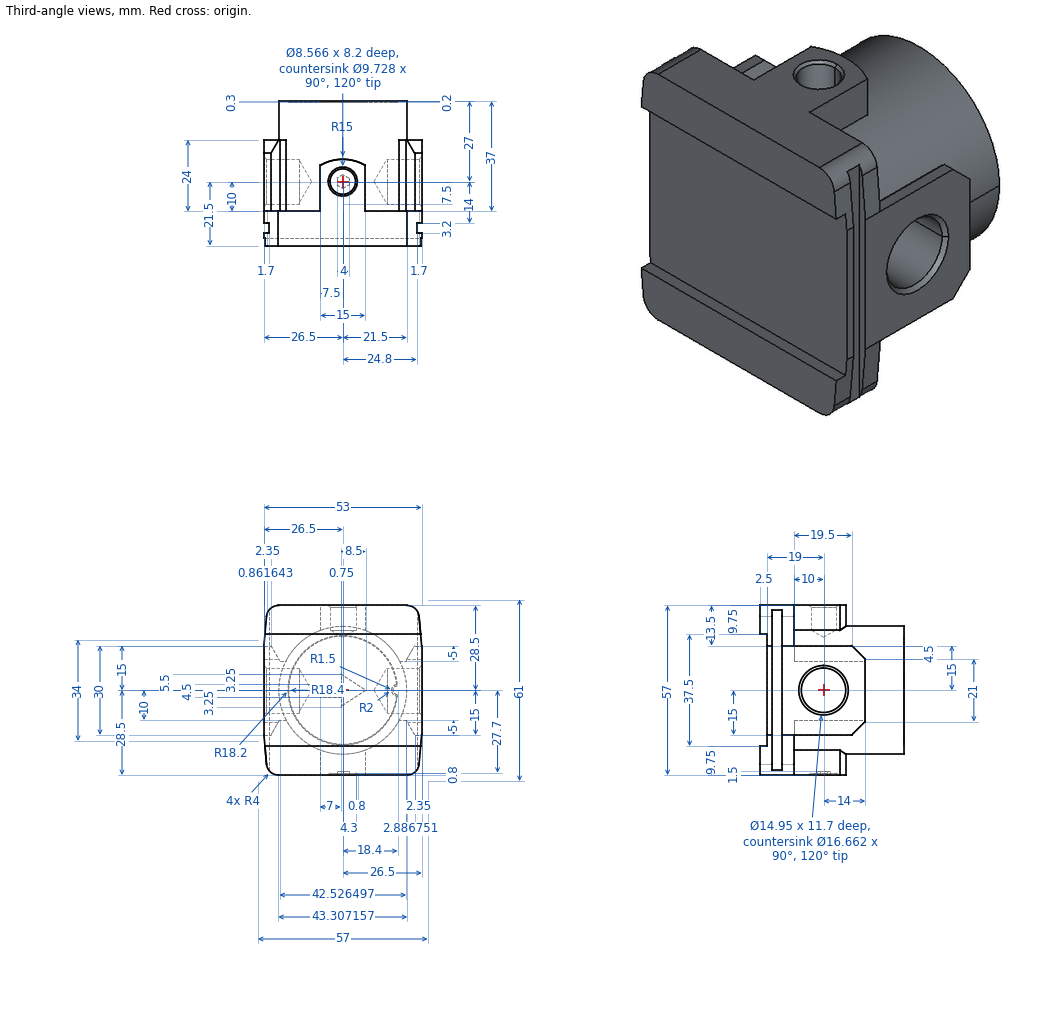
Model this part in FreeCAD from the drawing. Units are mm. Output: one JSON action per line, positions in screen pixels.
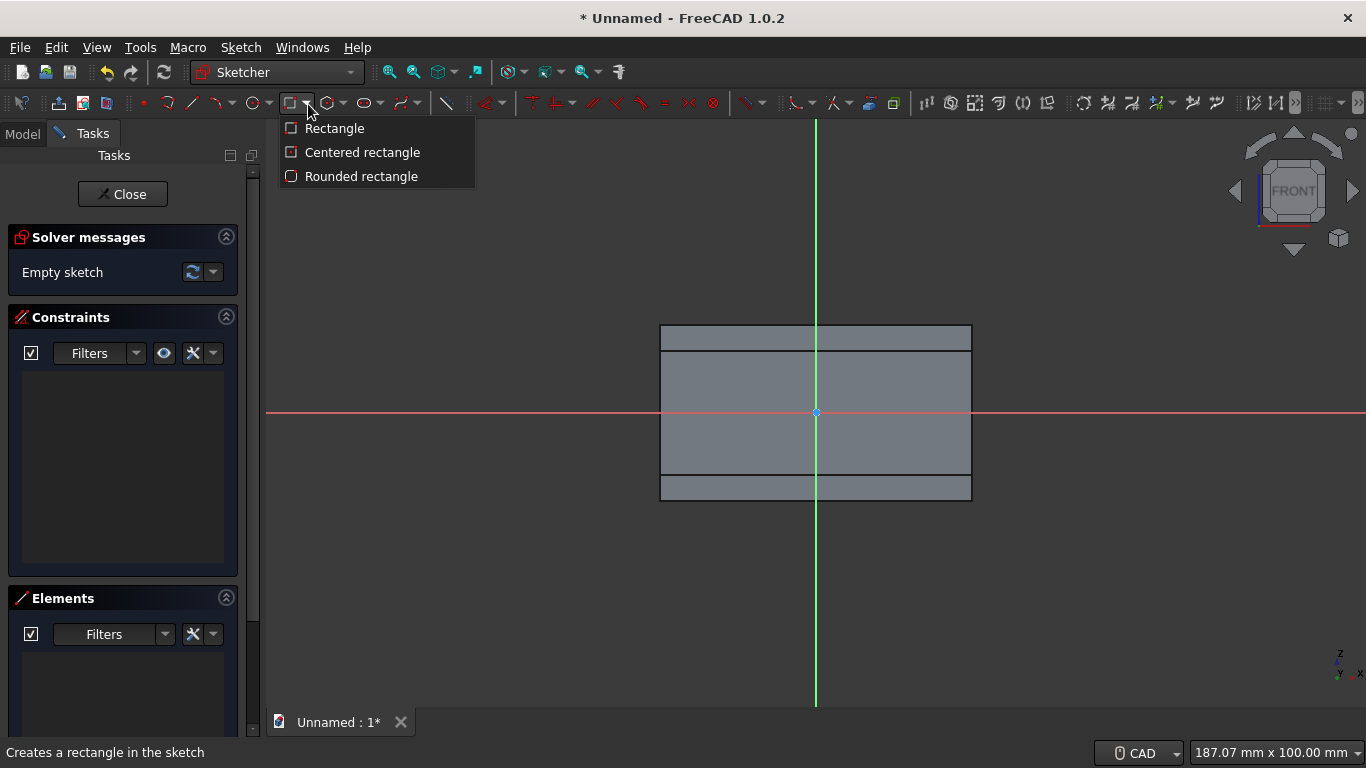
{"action": "left_click", "coordinate": [378, 152]}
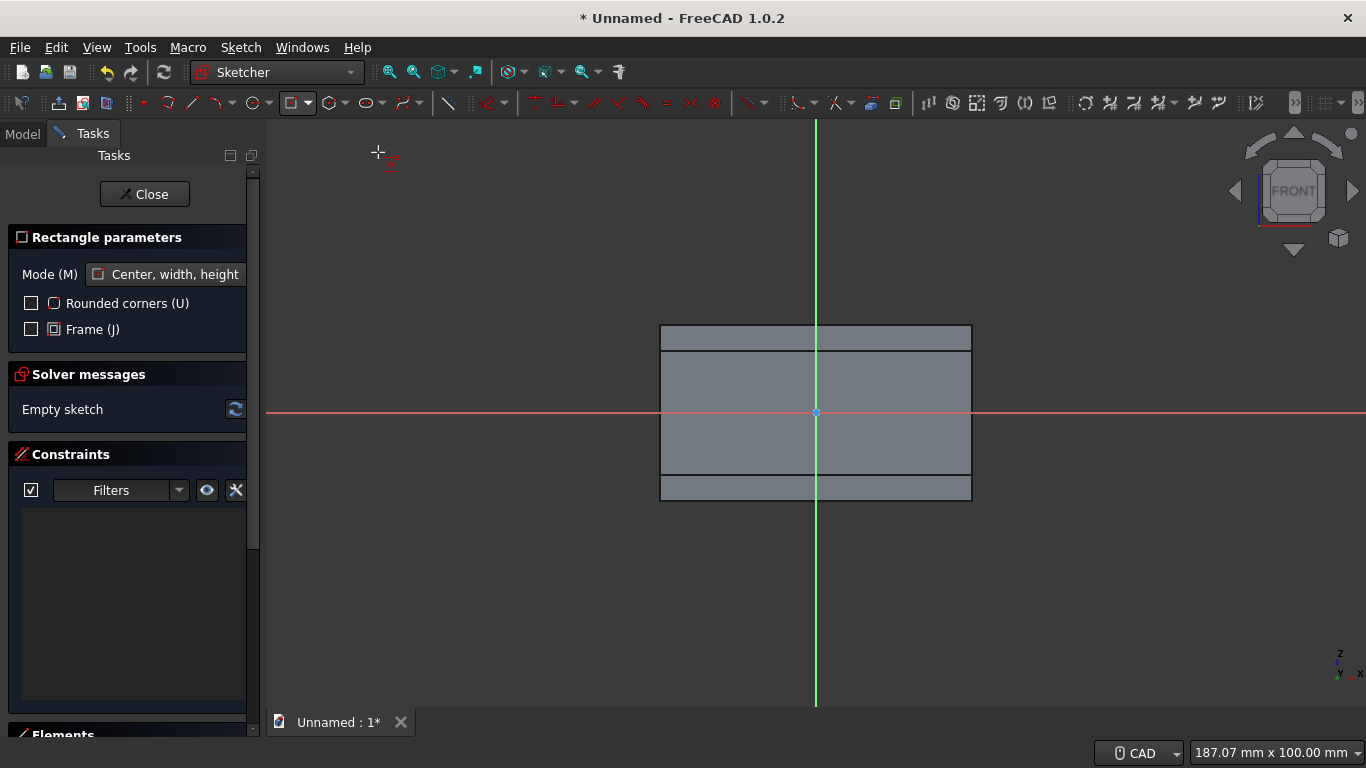
{"action": "left_click", "coordinate": [816, 413]}
{"action": "mouse_move", "coordinate": [984, 234]}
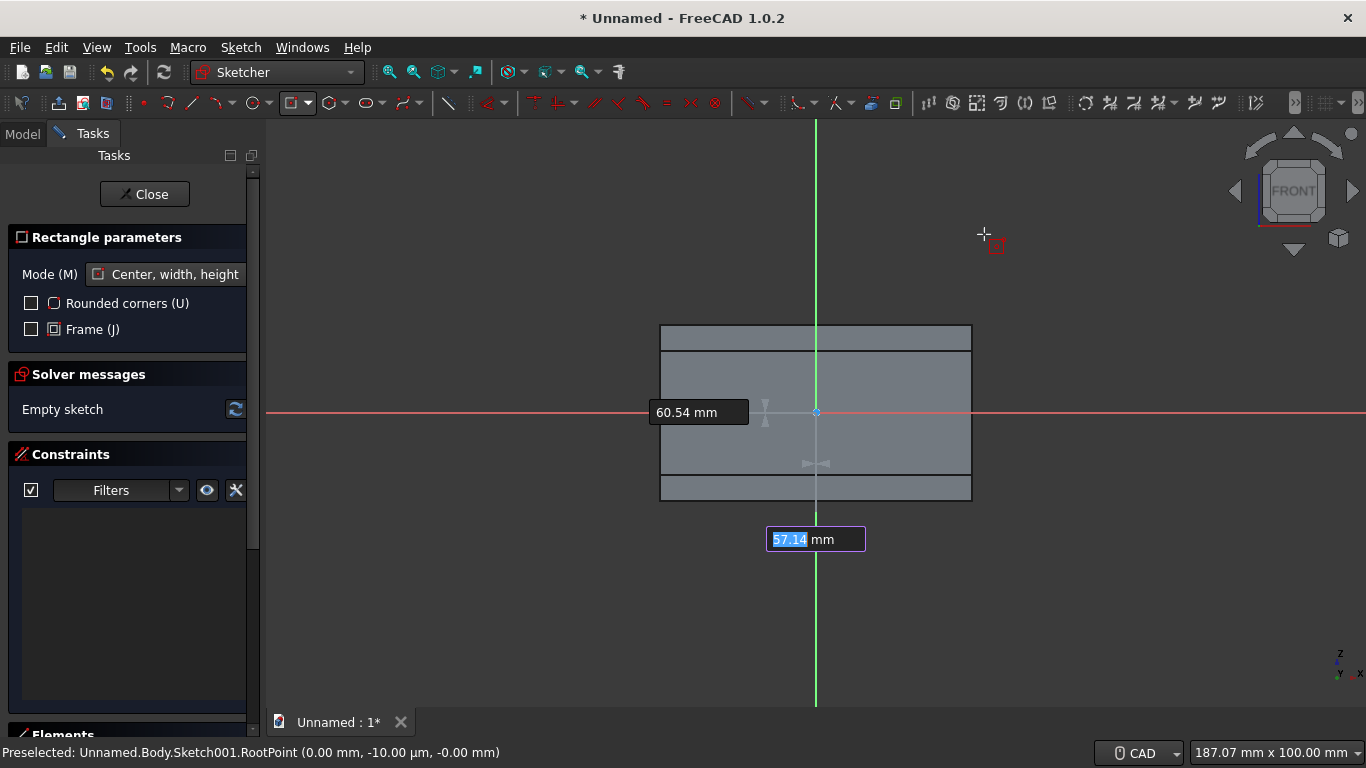
{"action": "type", "text": "57"}
{"action": "key", "text": "Tab"}
{"action": "type", "text": "61"}
{"action": "key", "text": "Return"}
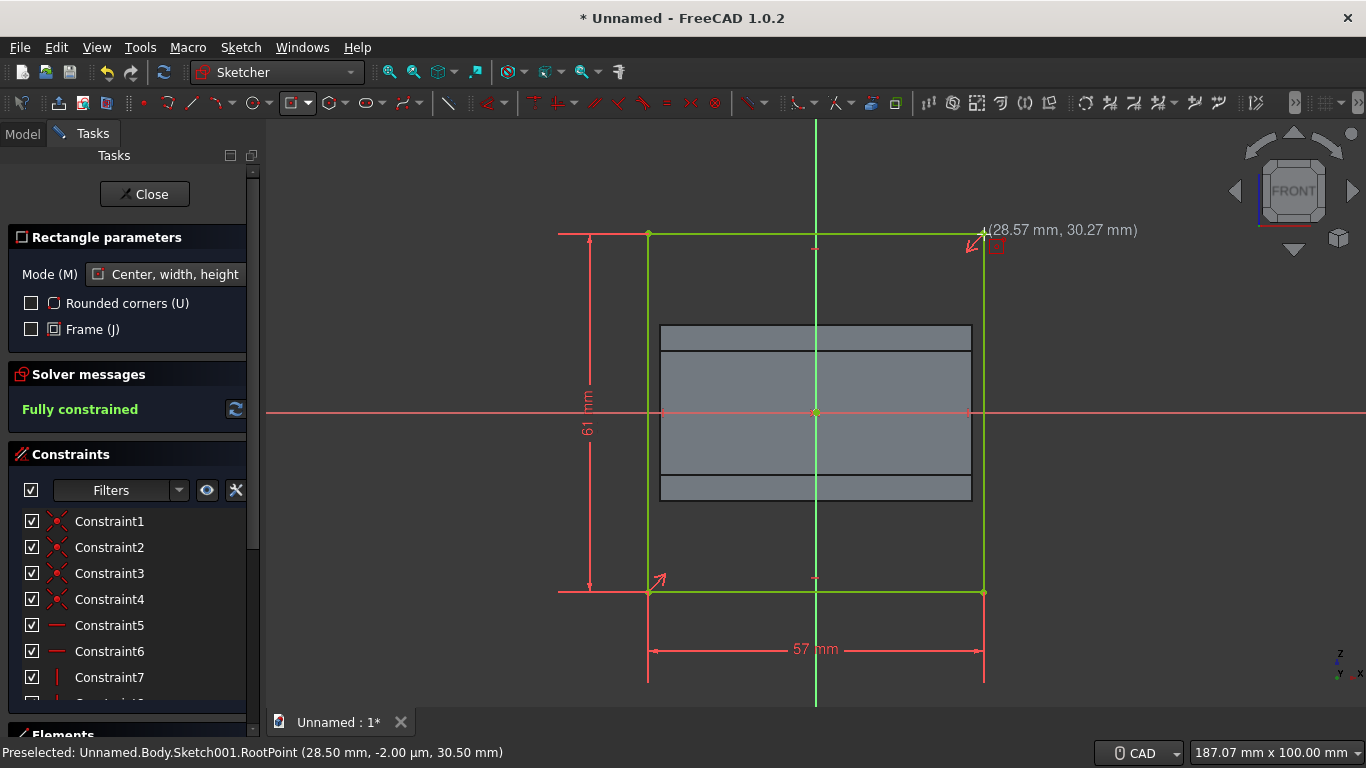
{"action": "left_click", "coordinate": [168, 104]}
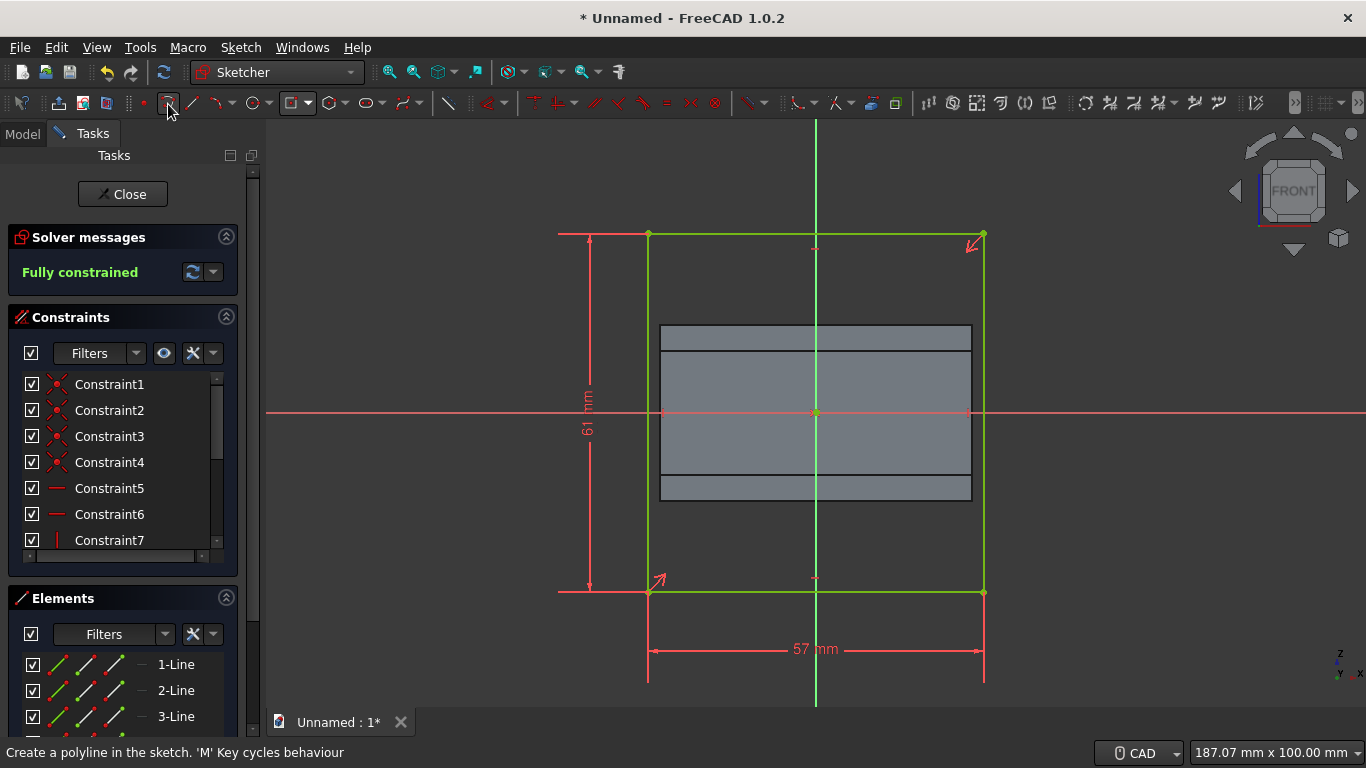
{"action": "left_click", "coordinate": [665, 267]}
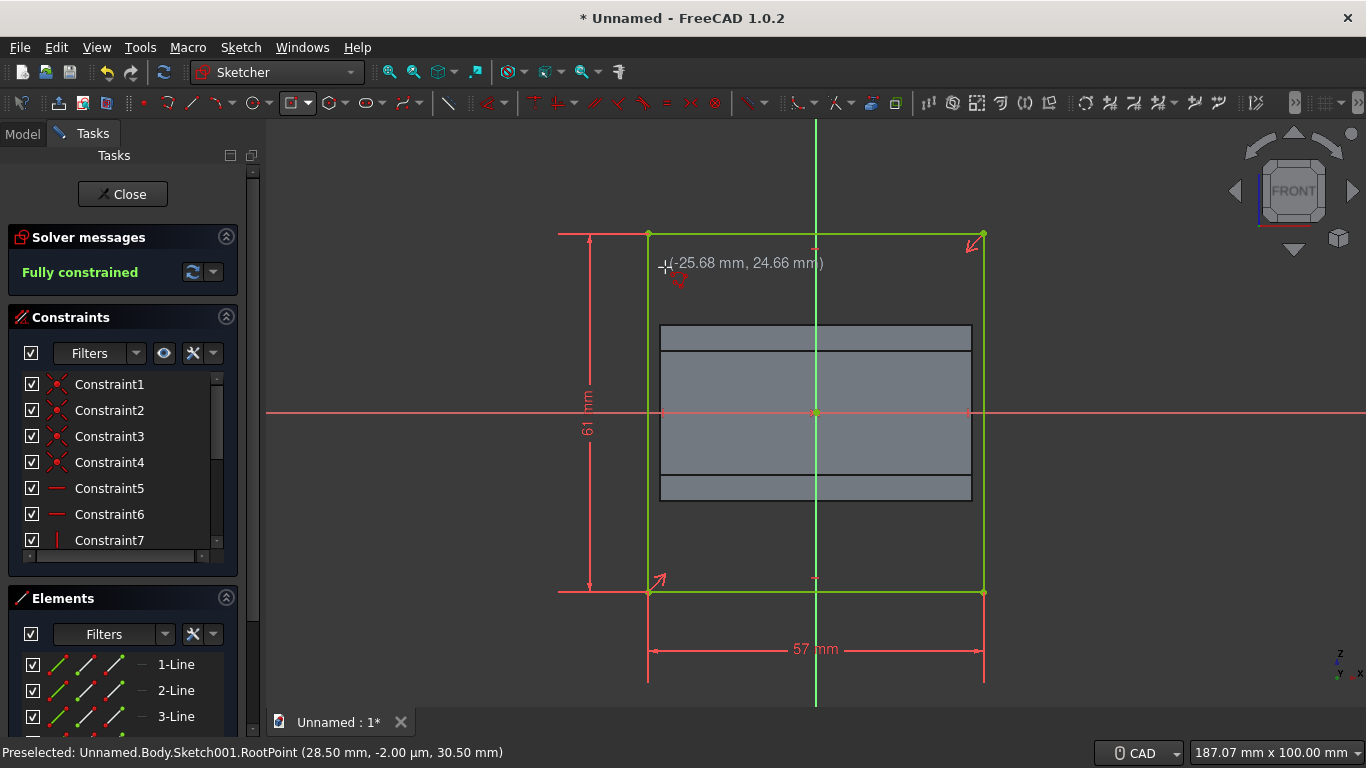
{"action": "scroll", "coordinate": [660, 325], "scroll_direction": "up", "scroll_amount": 2}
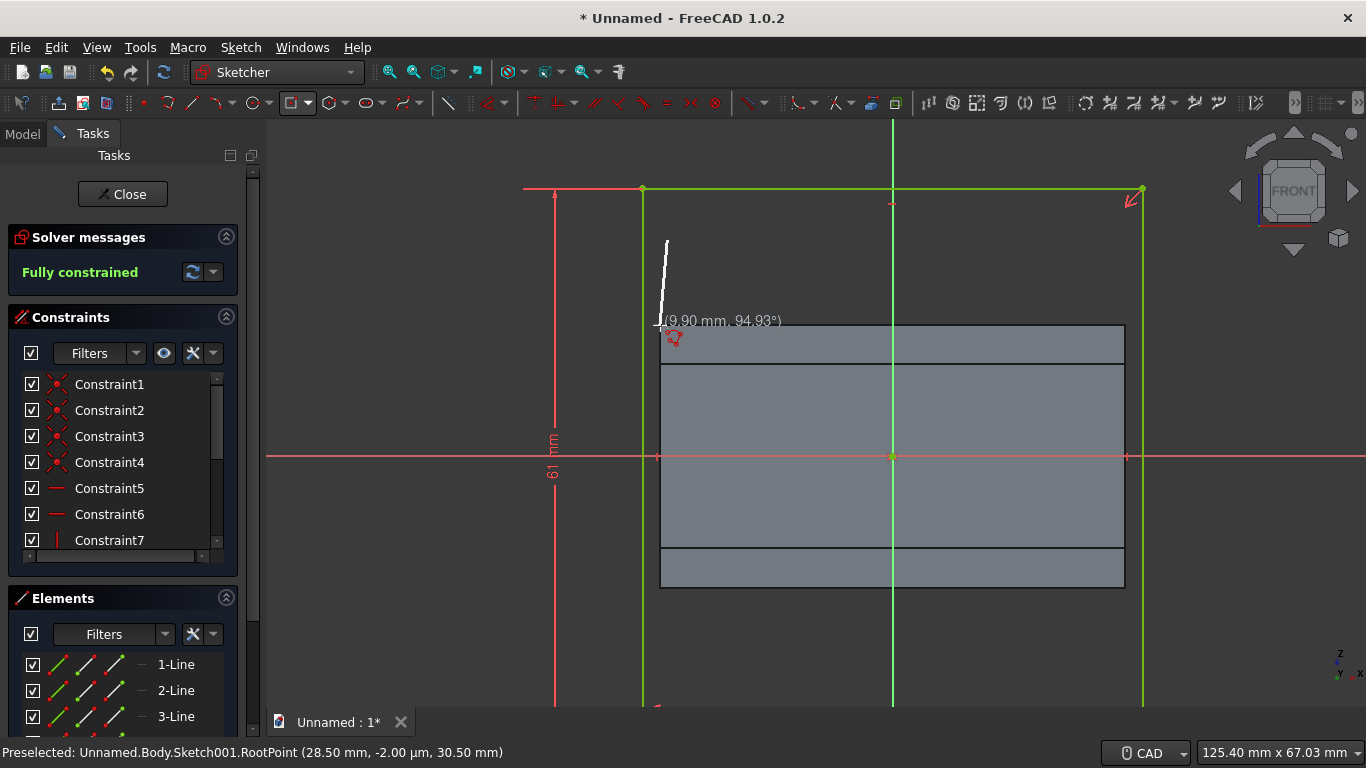
{"action": "left_click", "coordinate": [660, 325]}
{"action": "left_click", "coordinate": [660, 588]}
{"action": "left_click", "coordinate": [668, 674]}
{"action": "right_click", "coordinate": [668, 674]}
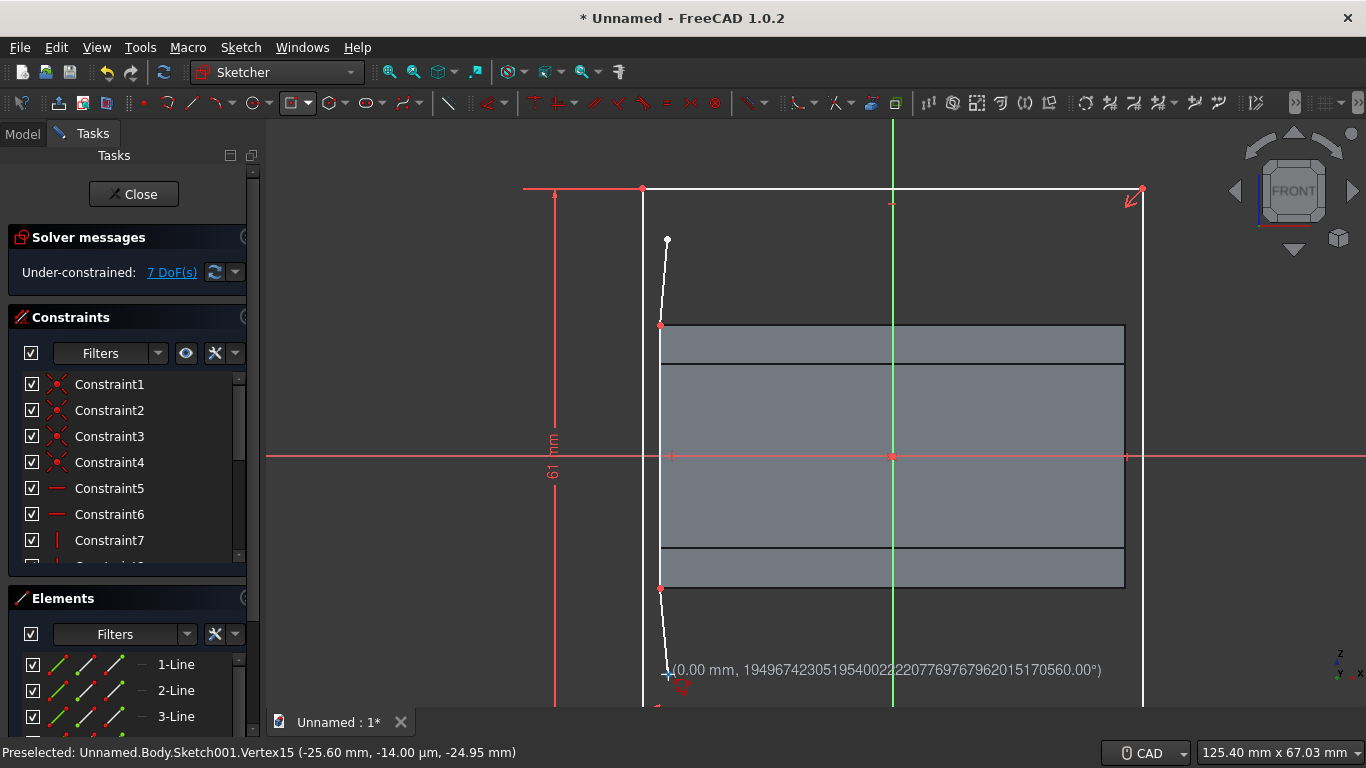
{"action": "left_click", "coordinate": [192, 104]}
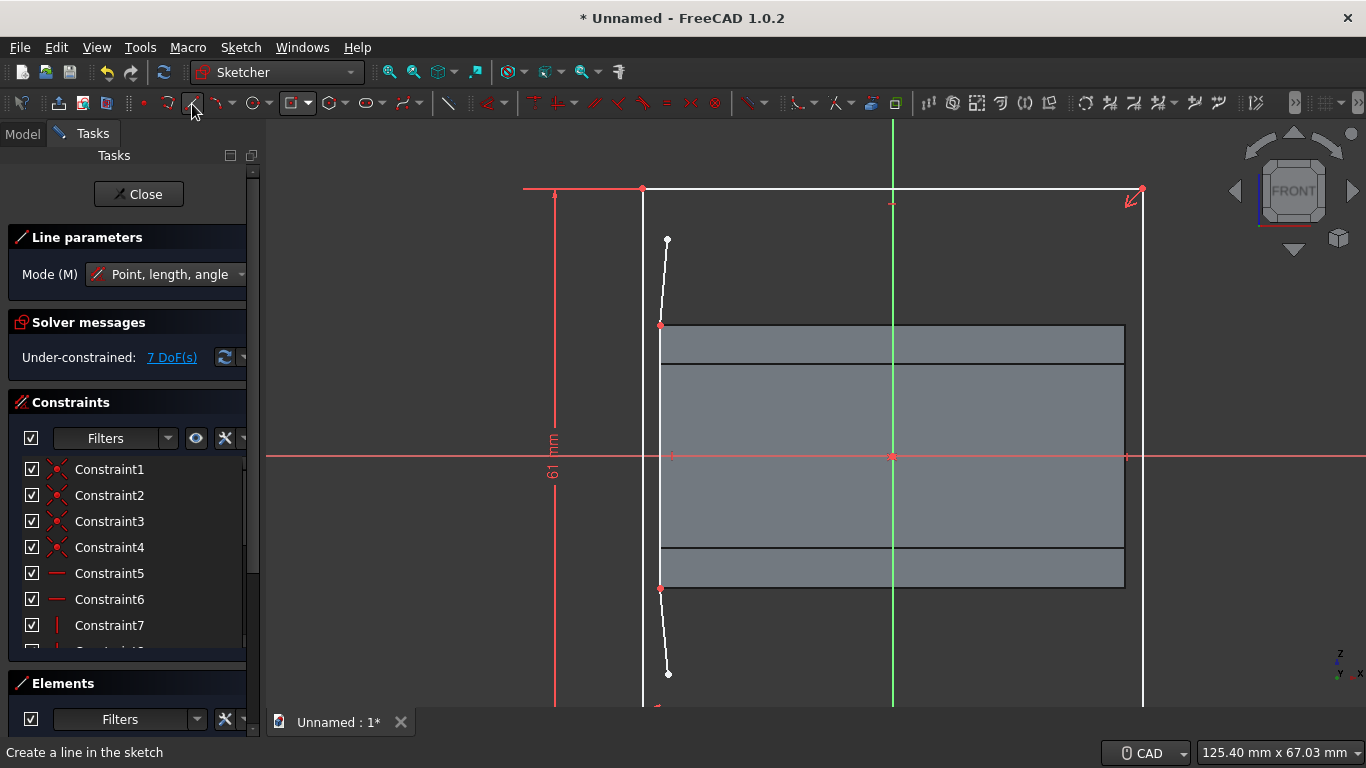
{"action": "scroll", "coordinate": [453, 325], "scroll_direction": "down", "scroll_amount": 2}